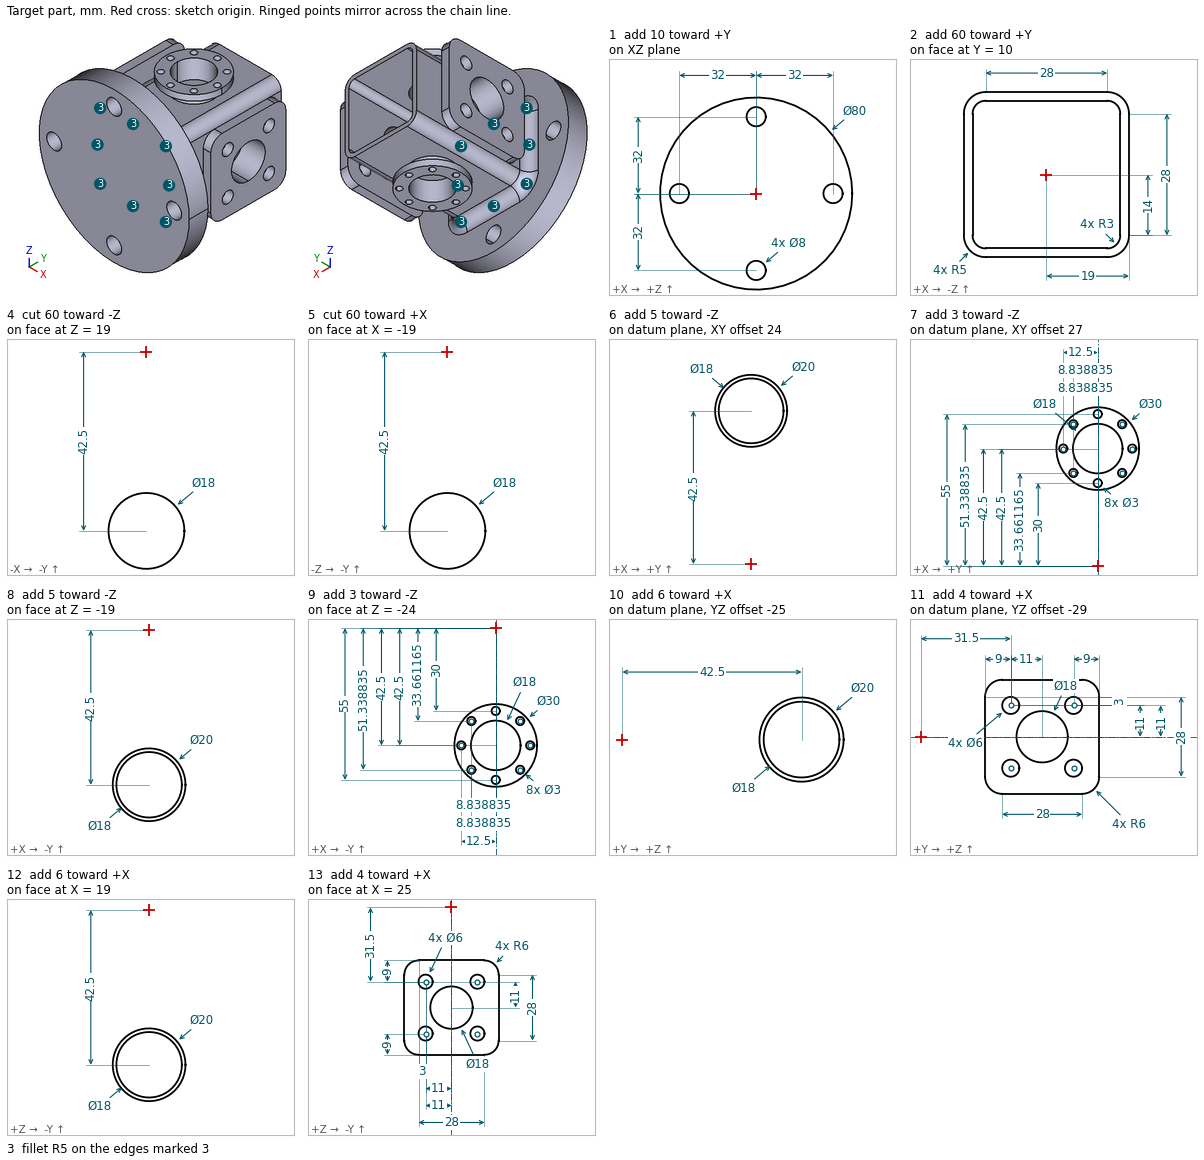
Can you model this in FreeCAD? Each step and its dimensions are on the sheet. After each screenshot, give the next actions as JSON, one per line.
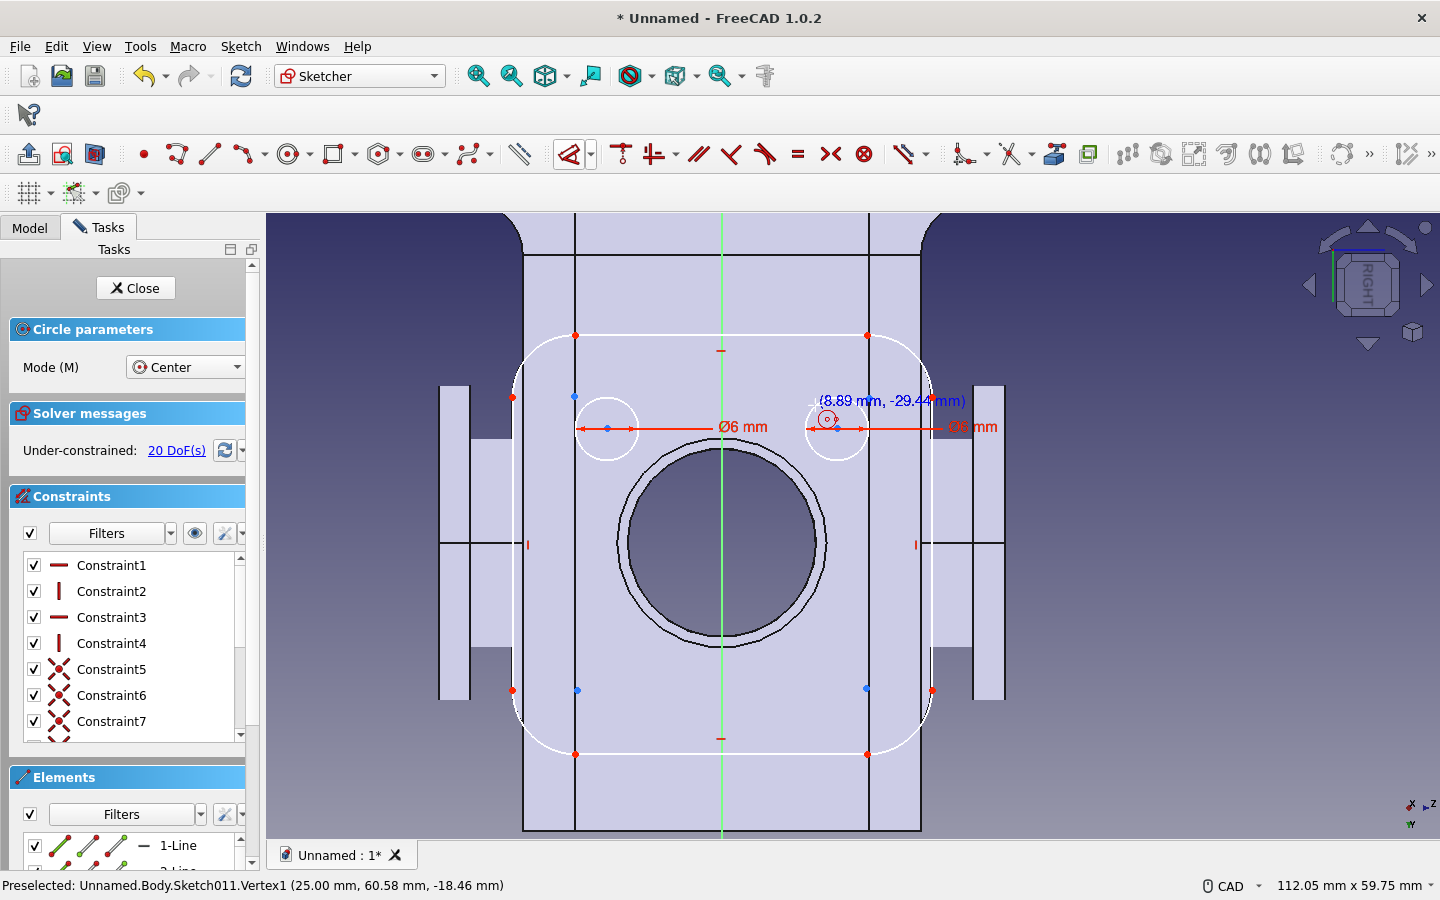
{"action": "left_click", "coordinate": [607, 658]}
{"action": "mouse_move", "coordinate": [629, 636]}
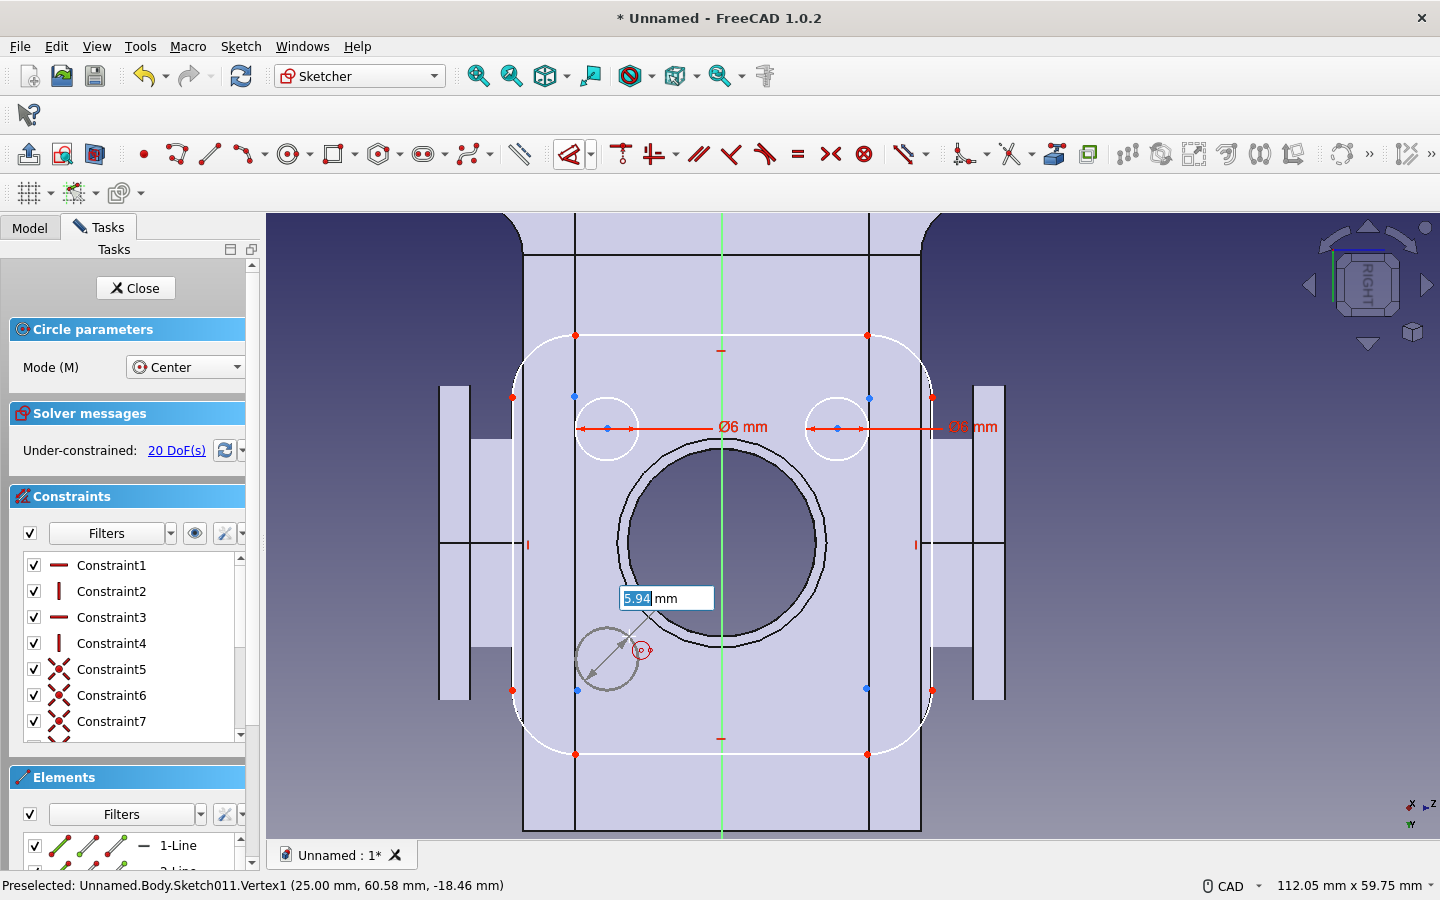
{"action": "type", "text": "6"}
{"action": "key", "text": "Return"}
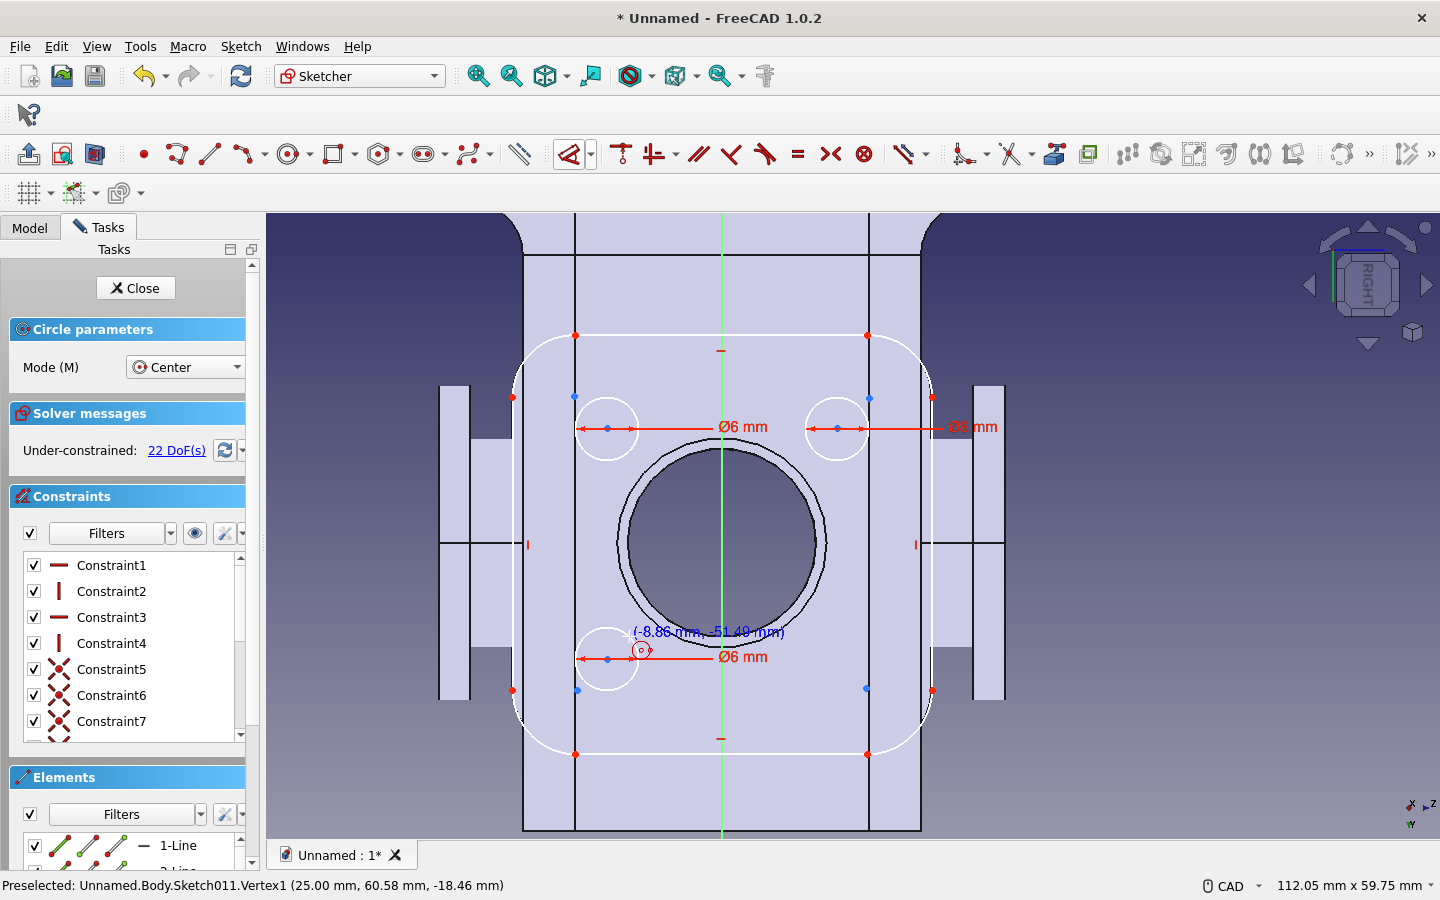
{"action": "left_click", "coordinate": [722, 543]}
{"action": "mouse_move", "coordinate": [789, 476]}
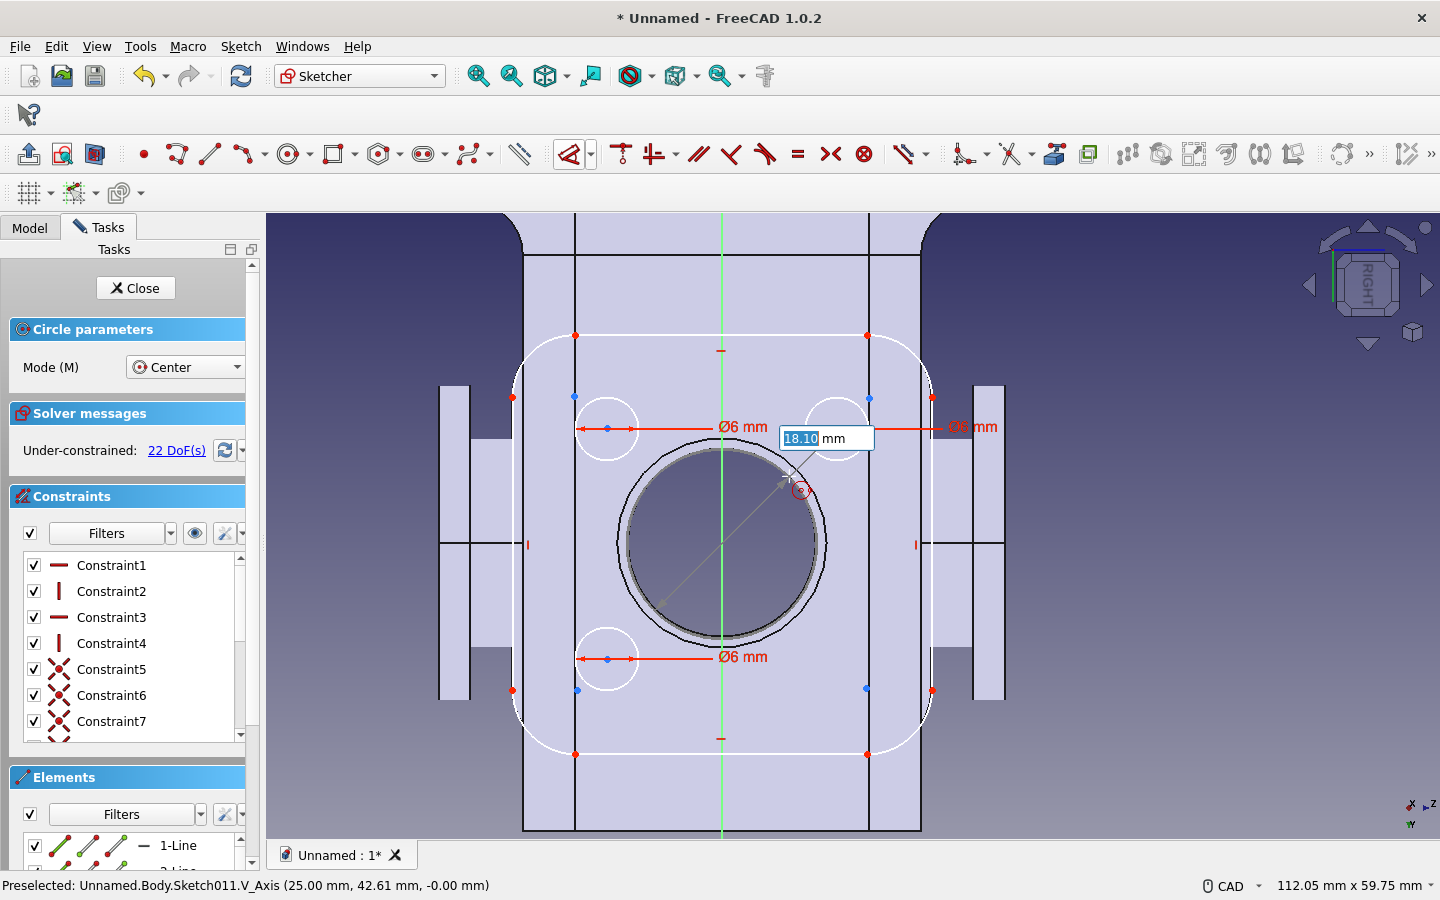
{"action": "type", "text": "18"}
{"action": "key", "text": "Return"}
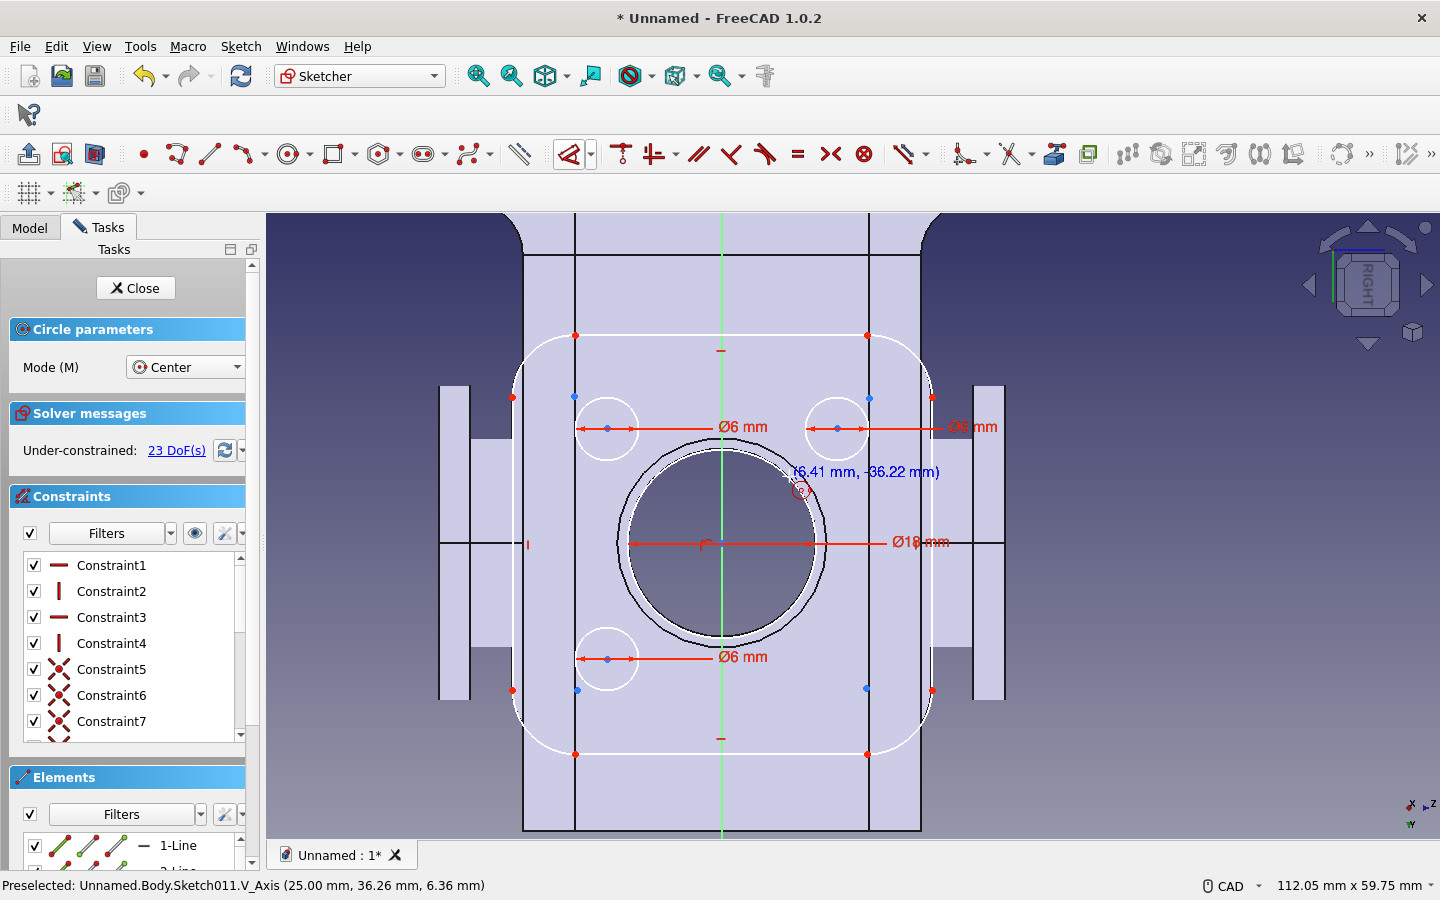
{"action": "left_click", "coordinate": [837, 658]}
{"action": "mouse_move", "coordinate": [859, 636]}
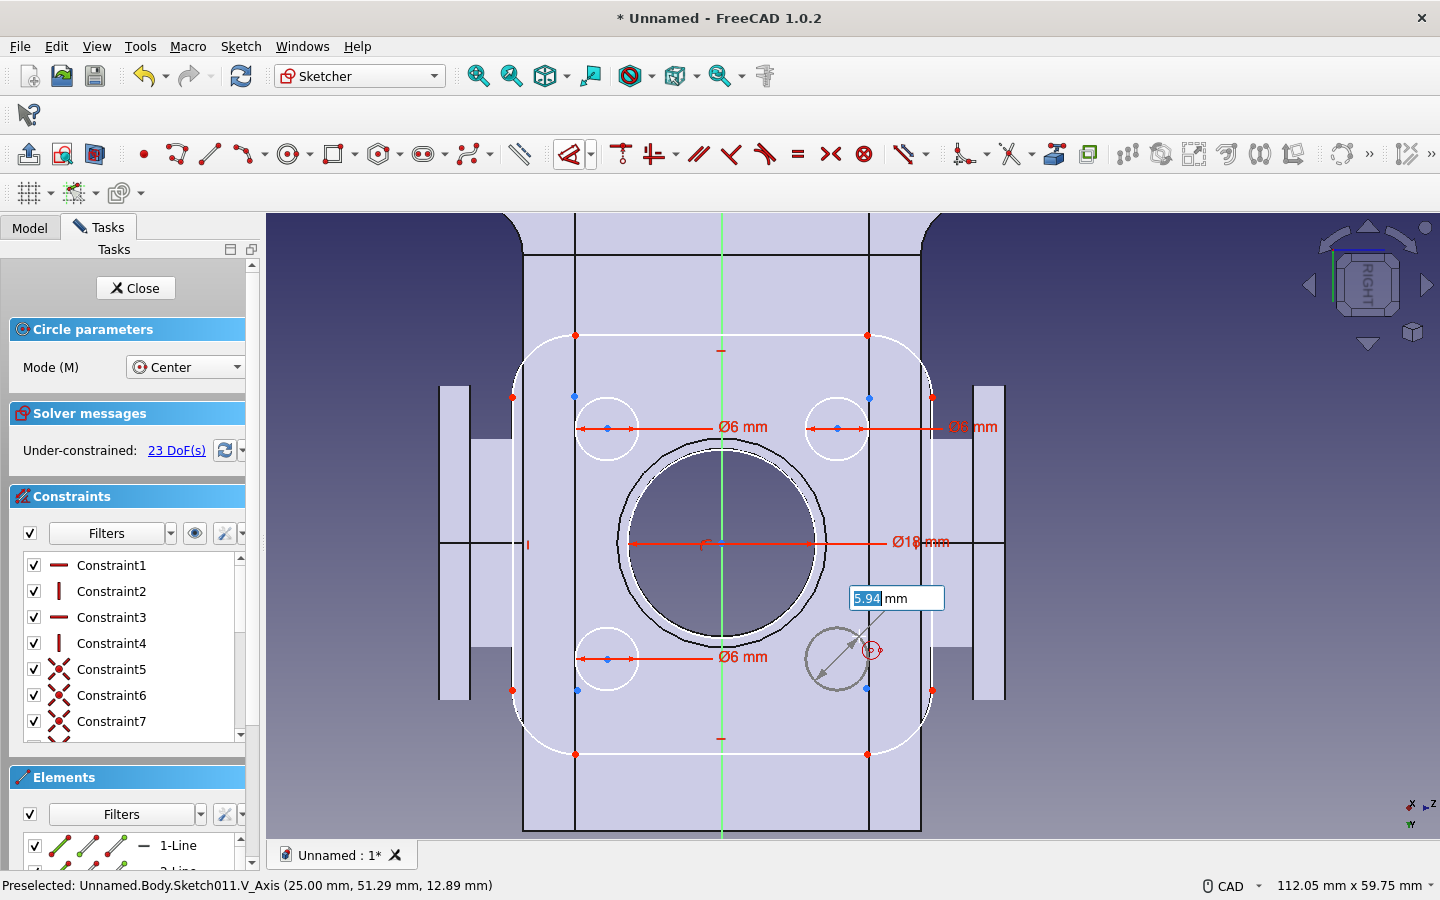
{"action": "type", "text": "6"}
{"action": "key", "text": "Return"}
{"action": "key", "text": "Escape"}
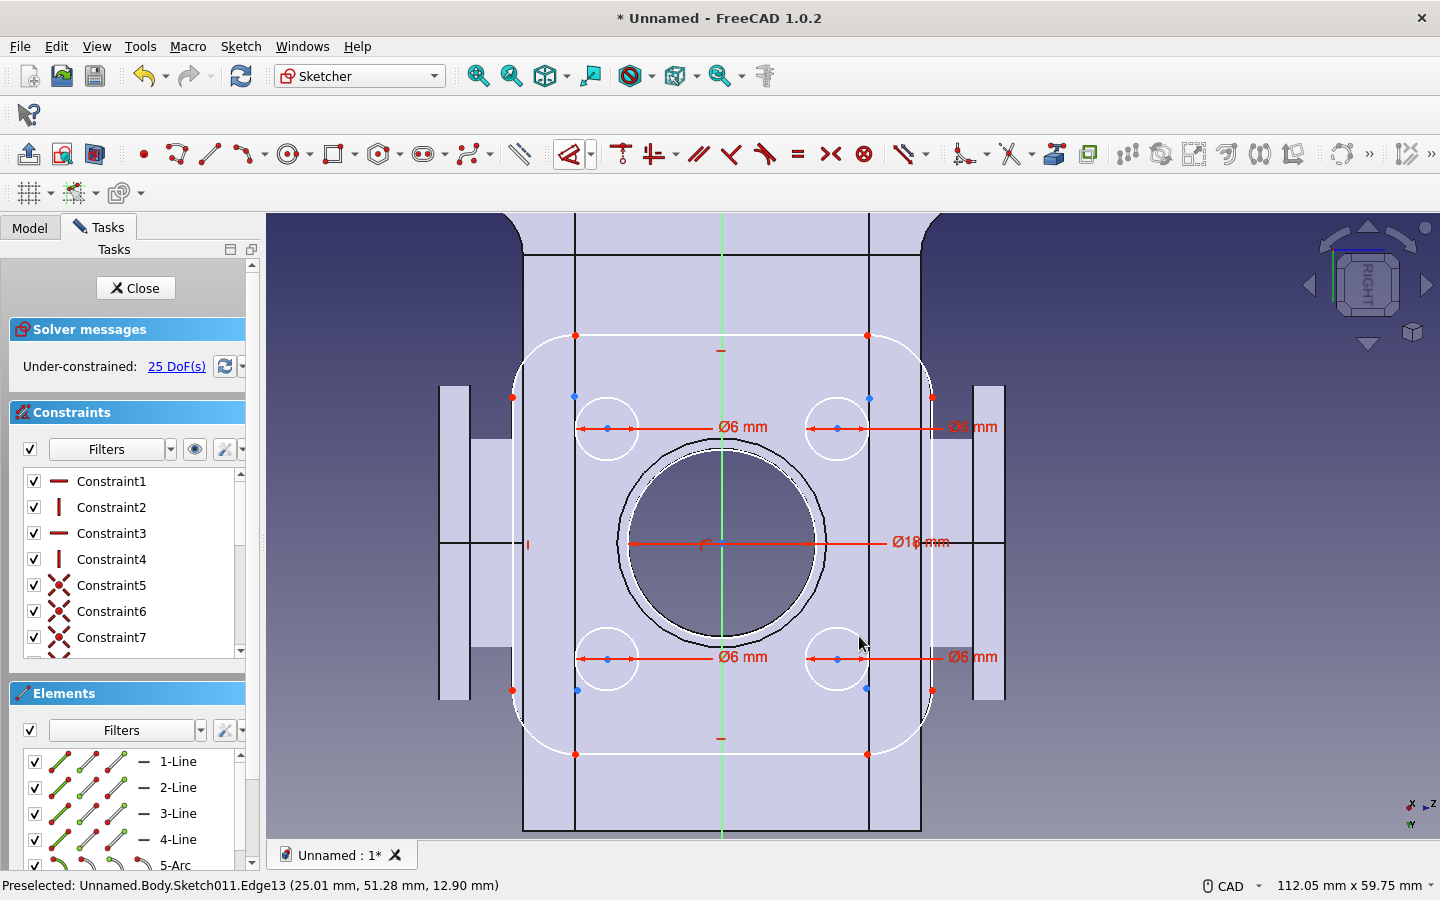
{"action": "left_click", "coordinate": [663, 754]}